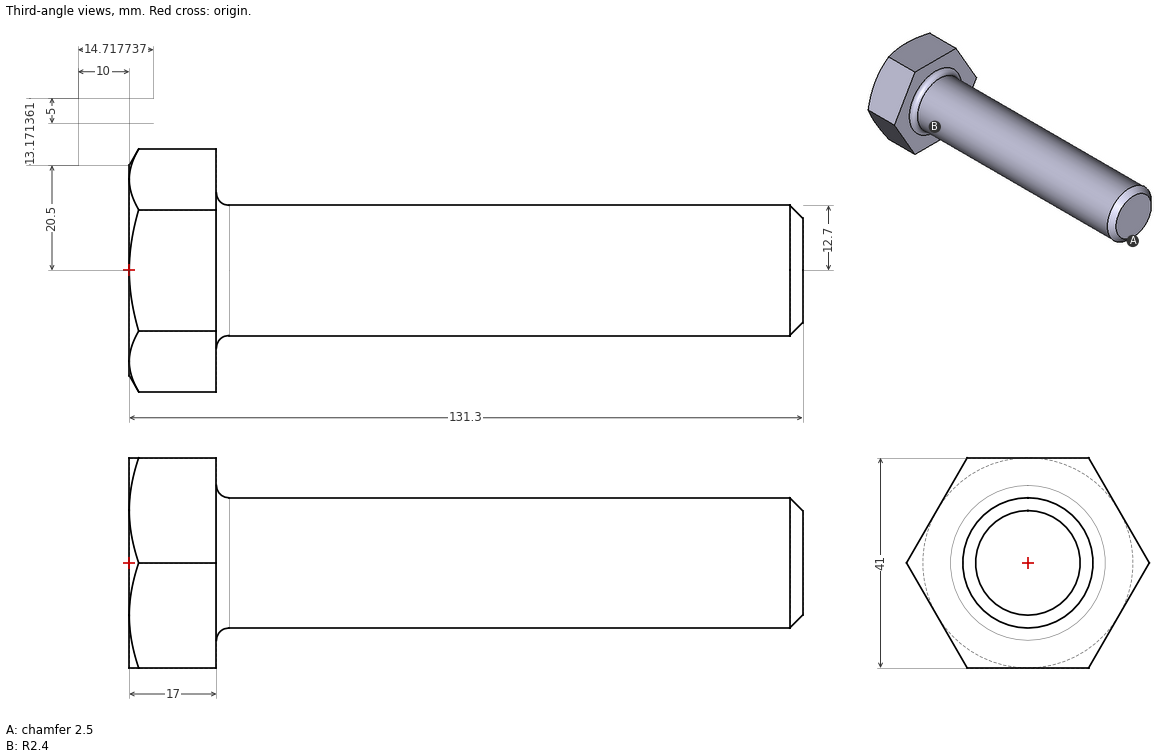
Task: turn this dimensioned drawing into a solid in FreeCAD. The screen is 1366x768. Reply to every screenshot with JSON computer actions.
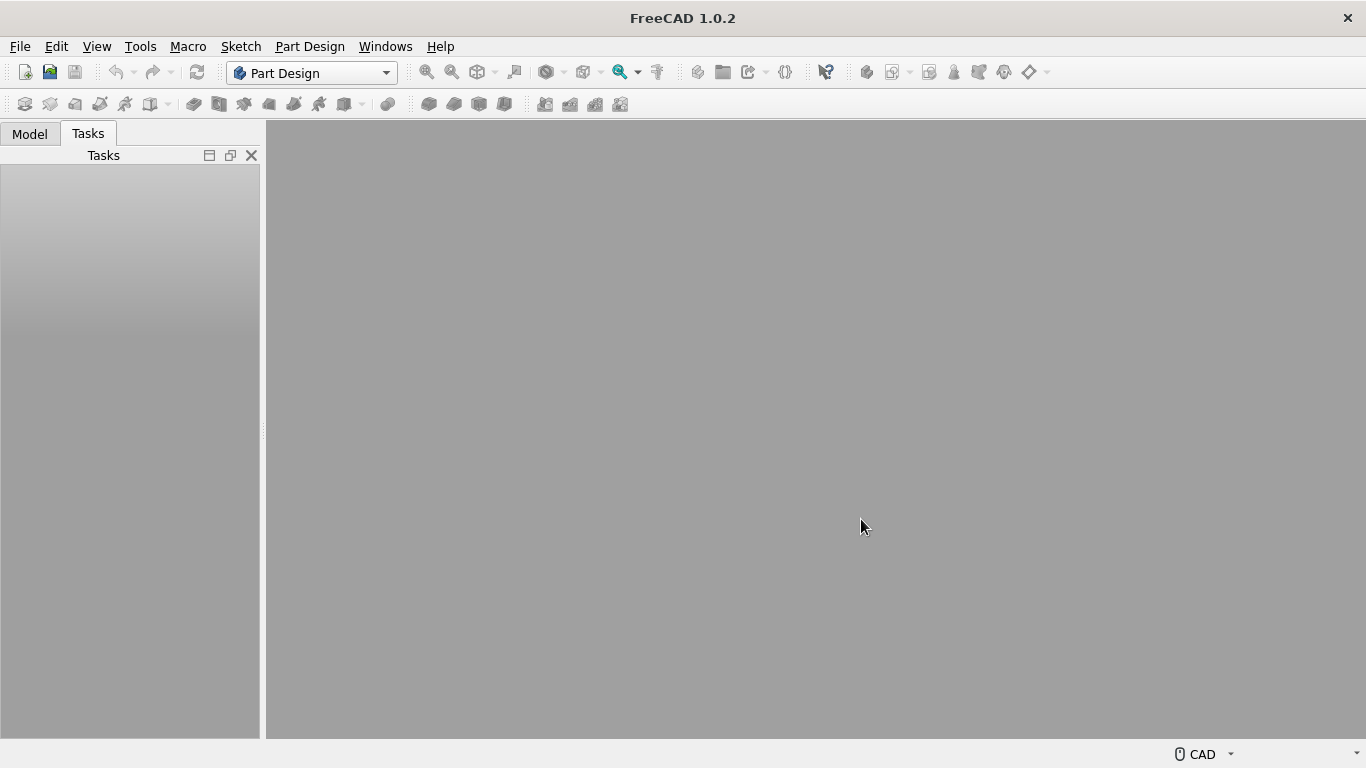
{"action": "key", "text": "ctrl+n"}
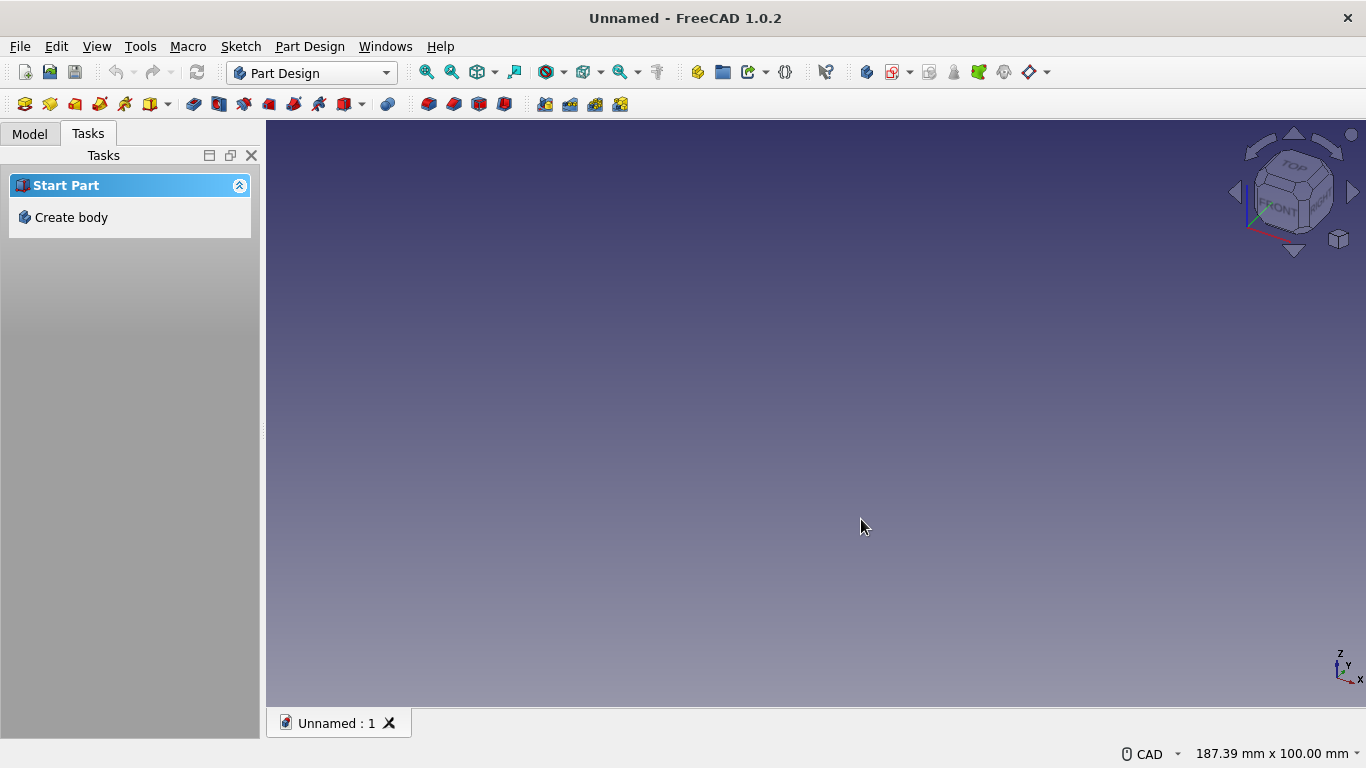
{"action": "left_click", "coordinate": [892, 72]}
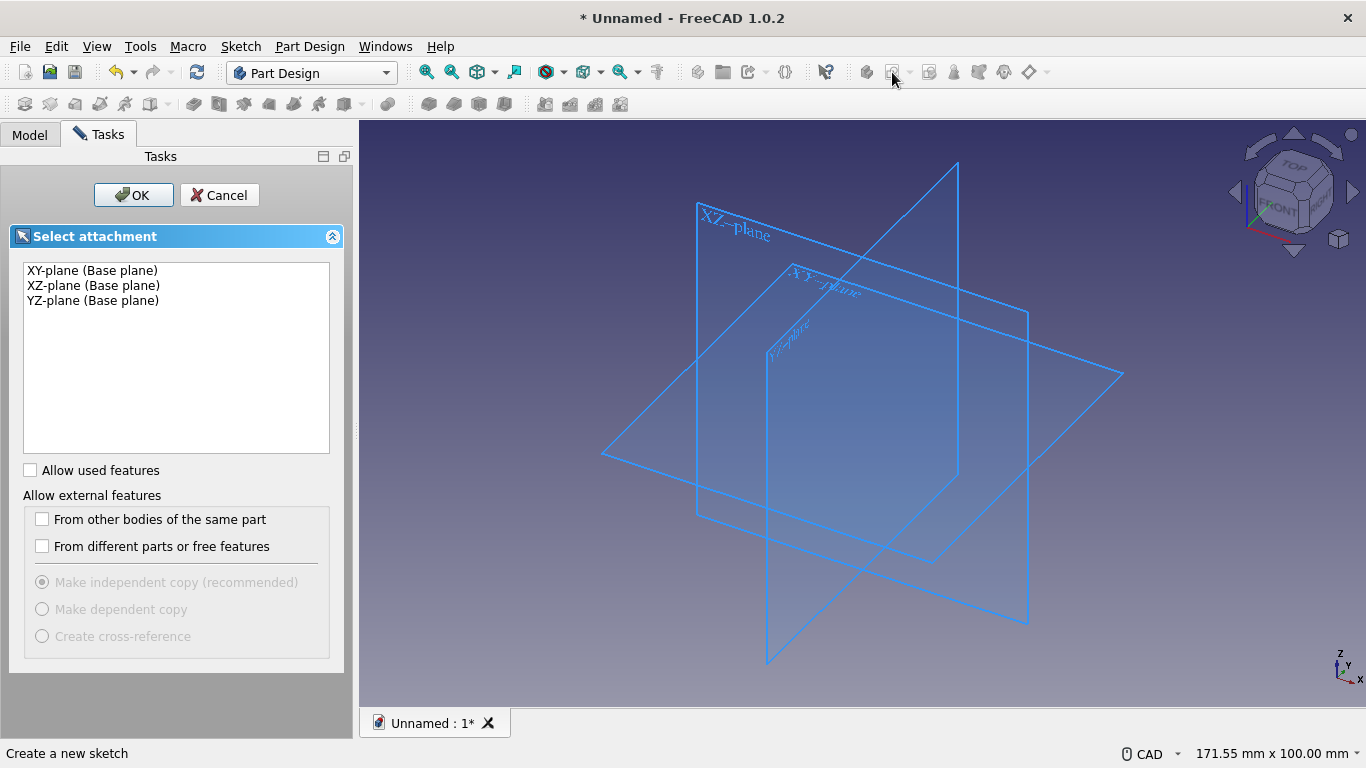
{"action": "left_click", "coordinate": [84, 300]}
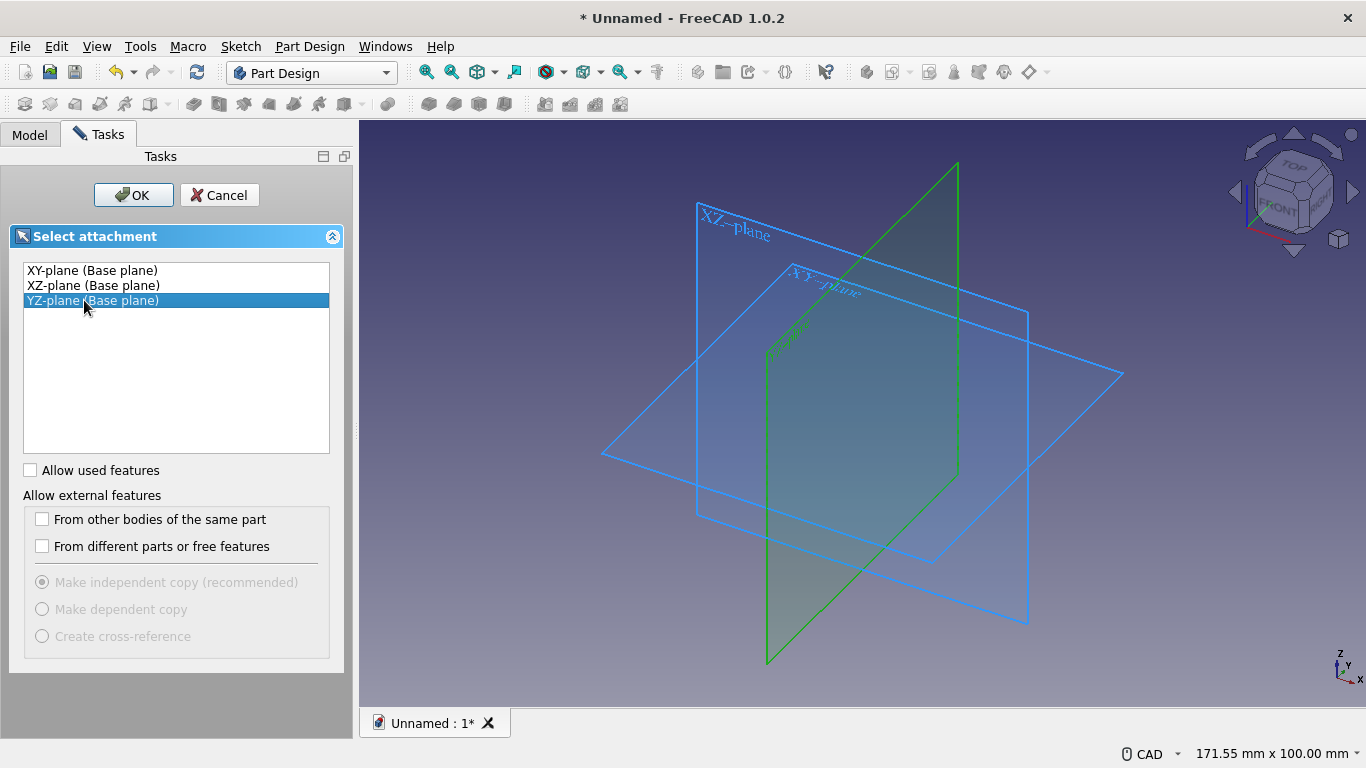
{"action": "left_click", "coordinate": [134, 195]}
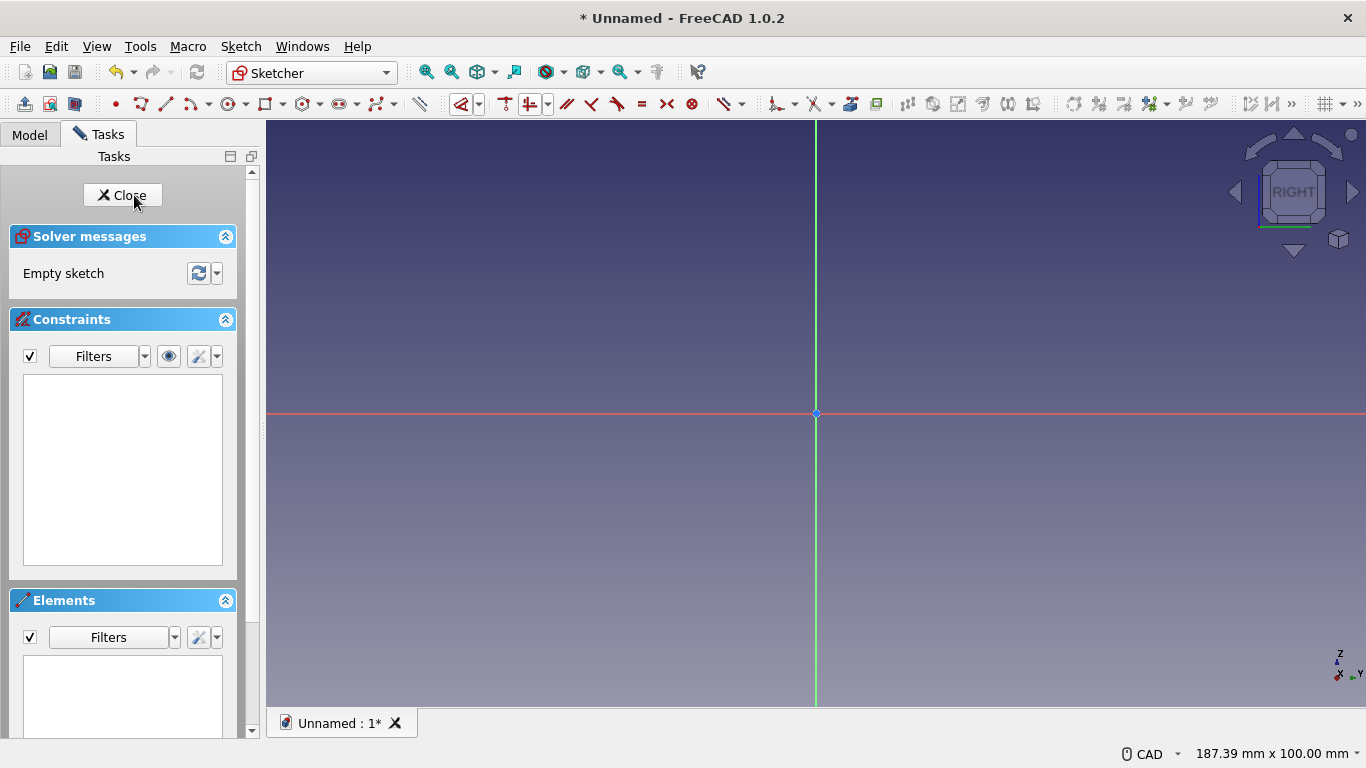
{"action": "scroll", "coordinate": [955, 413], "scroll_direction": "up", "scroll_amount": 2}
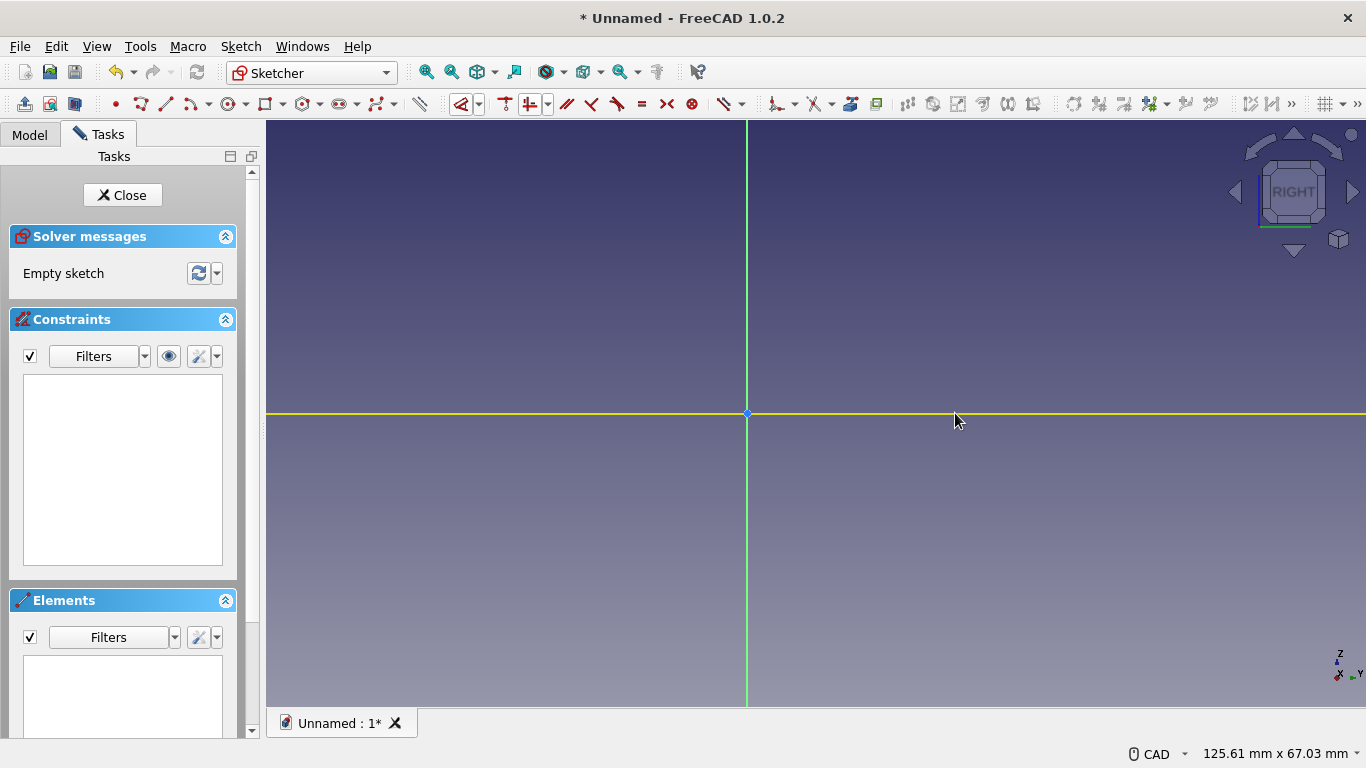
{"action": "key", "text": "g p 6"}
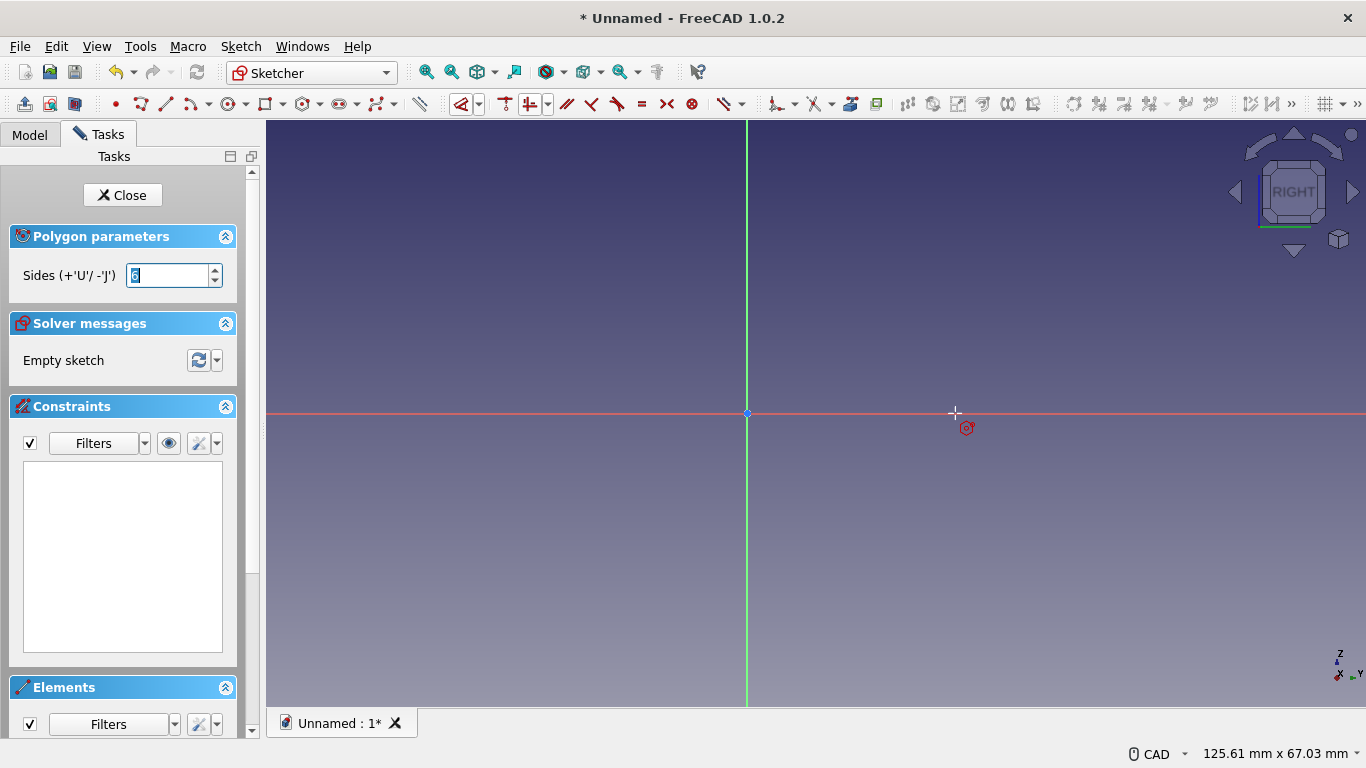
{"action": "left_click", "coordinate": [747, 414]}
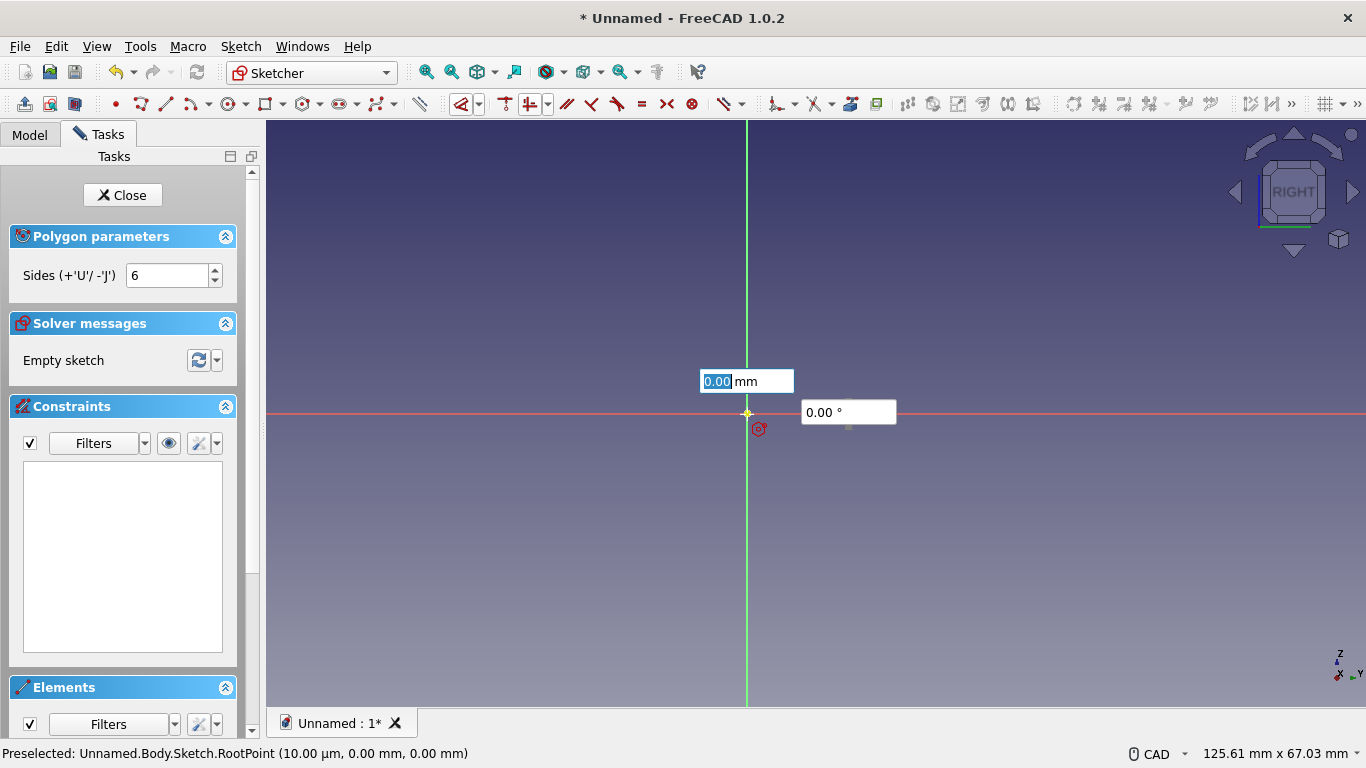
{"action": "left_click", "coordinate": [955, 414]}
{"action": "right_click", "coordinate": [955, 414]}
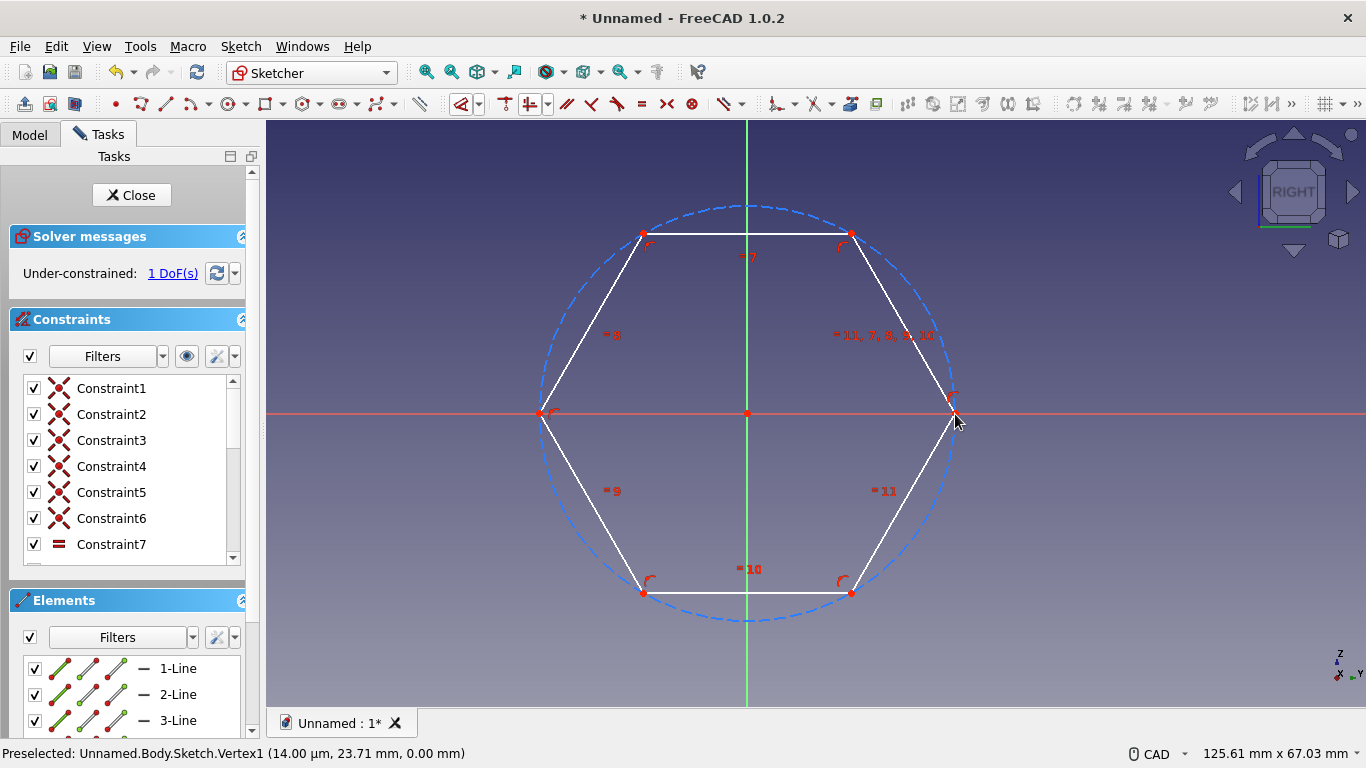
{"action": "key", "text": "d"}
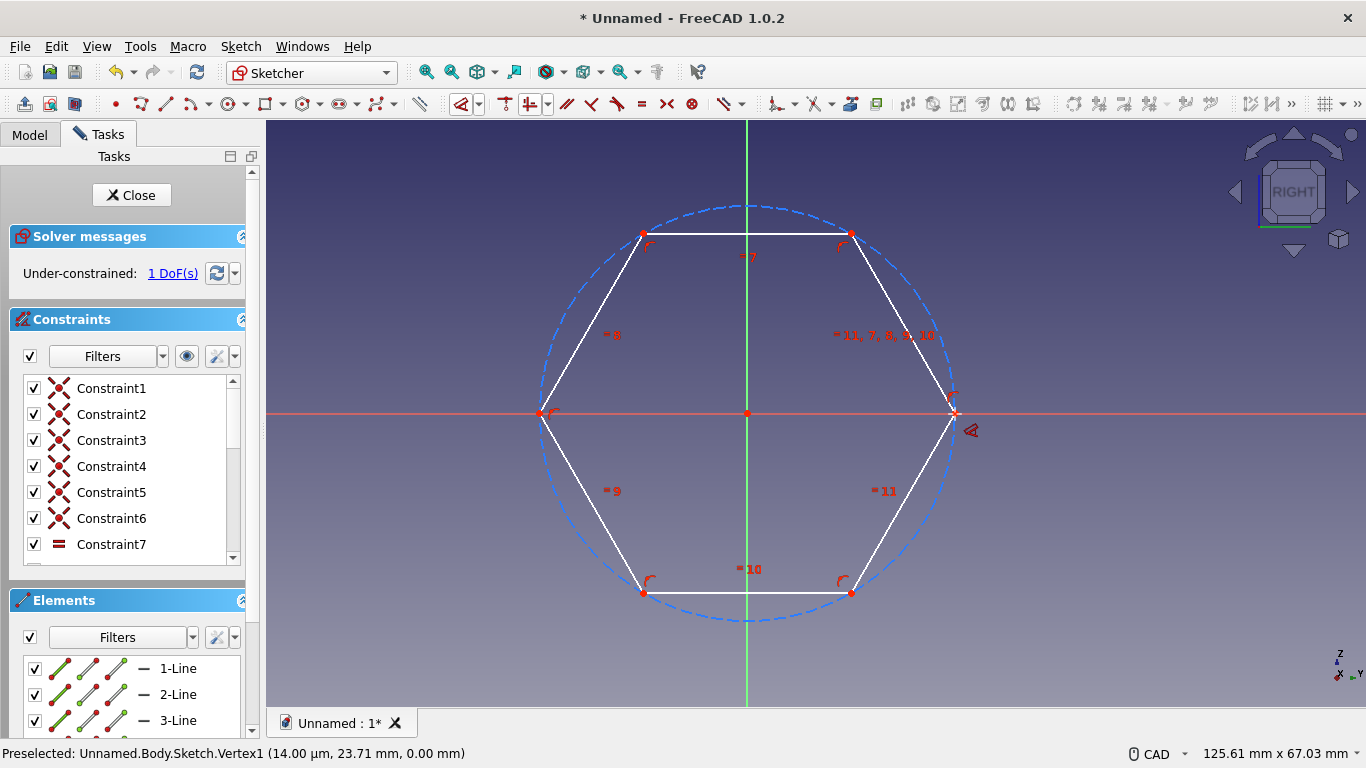
{"action": "left_click", "coordinate": [643, 593]}